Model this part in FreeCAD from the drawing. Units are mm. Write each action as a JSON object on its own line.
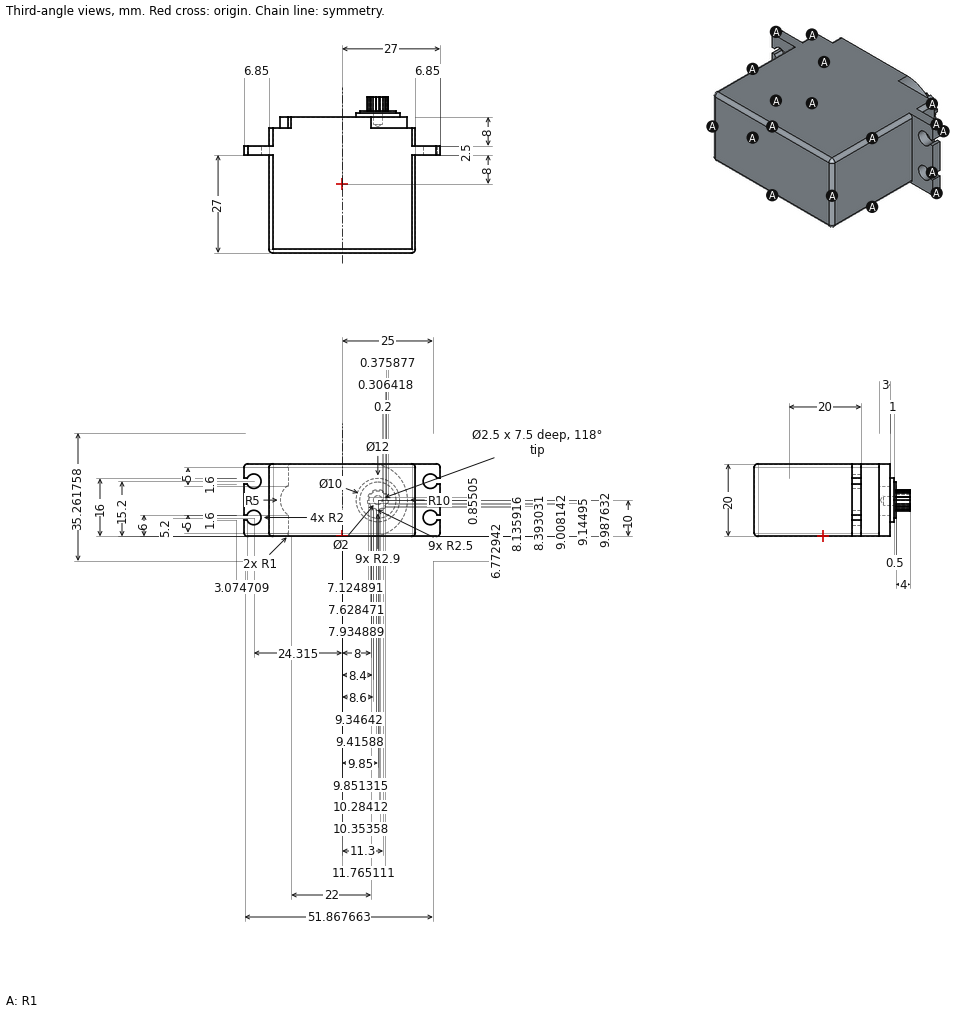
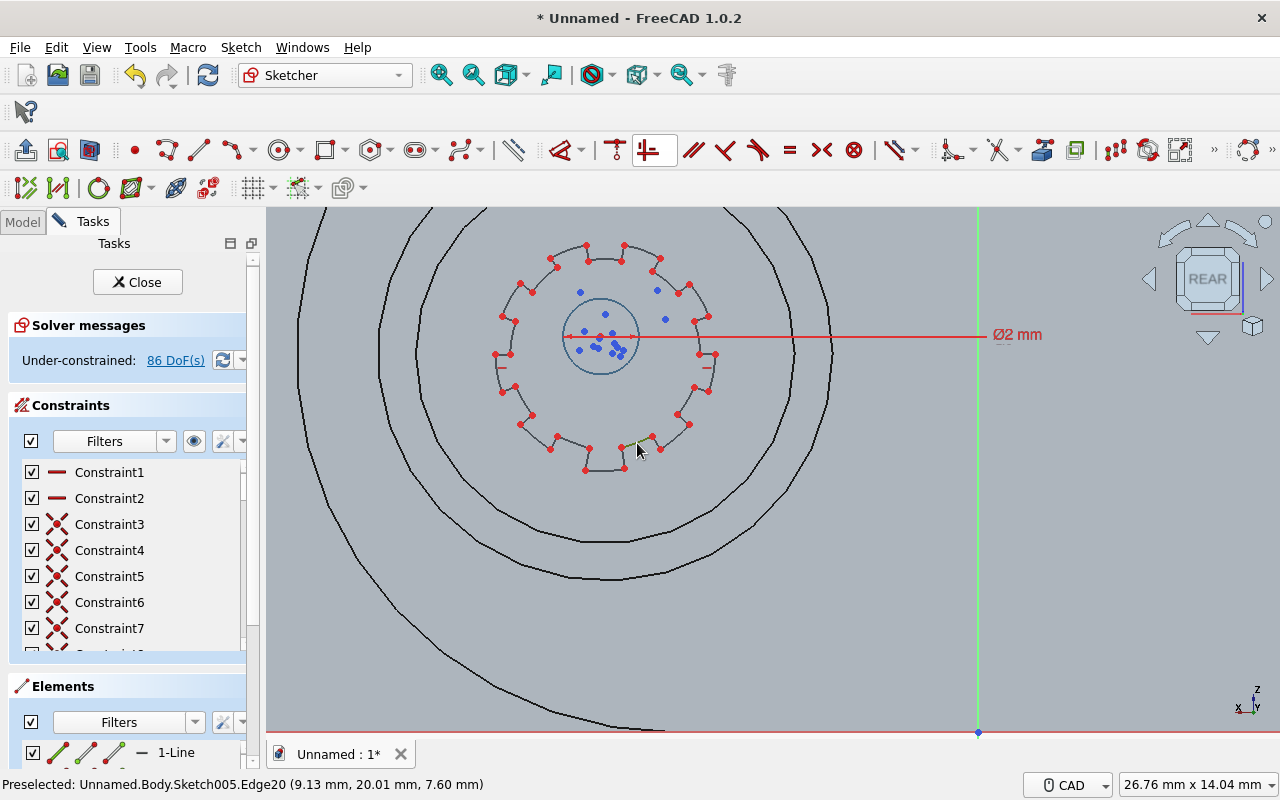
{"action": "left_click", "coordinate": [616, 150]}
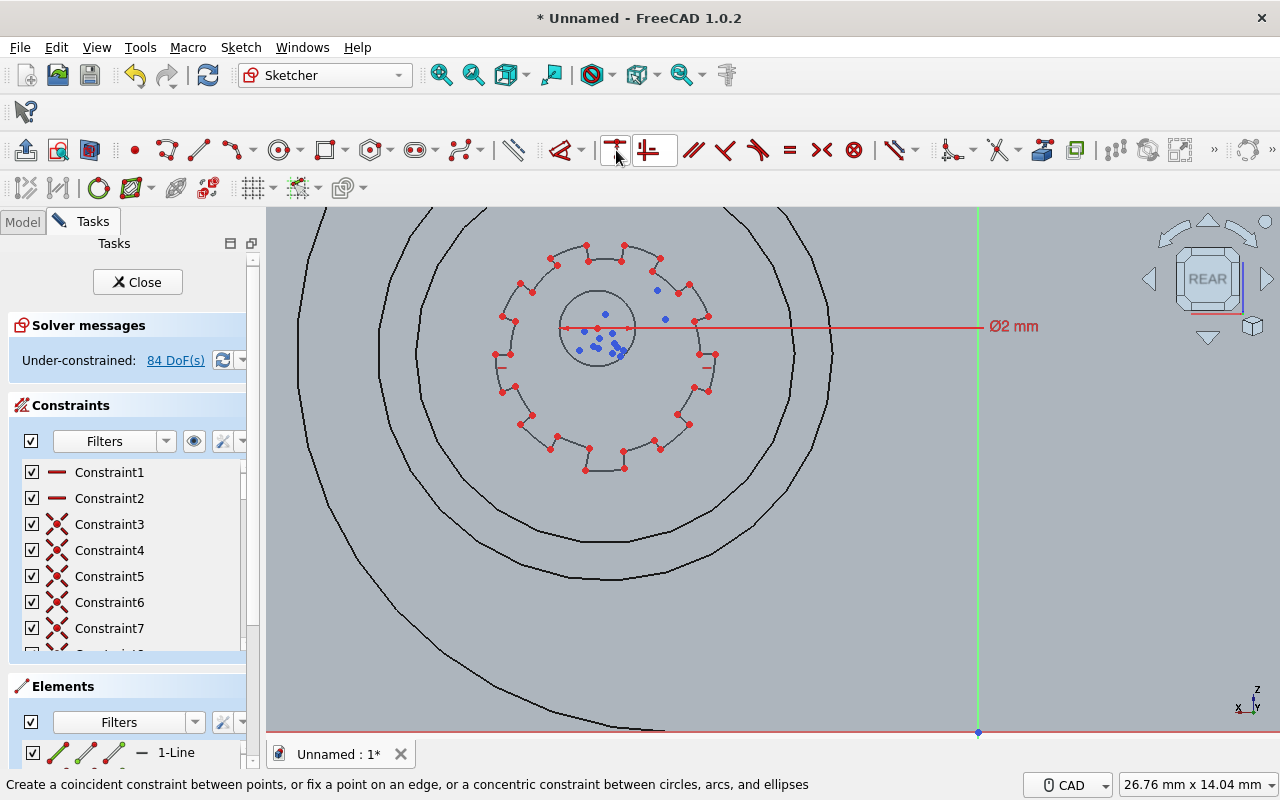
{"action": "left_click", "coordinate": [624, 302]}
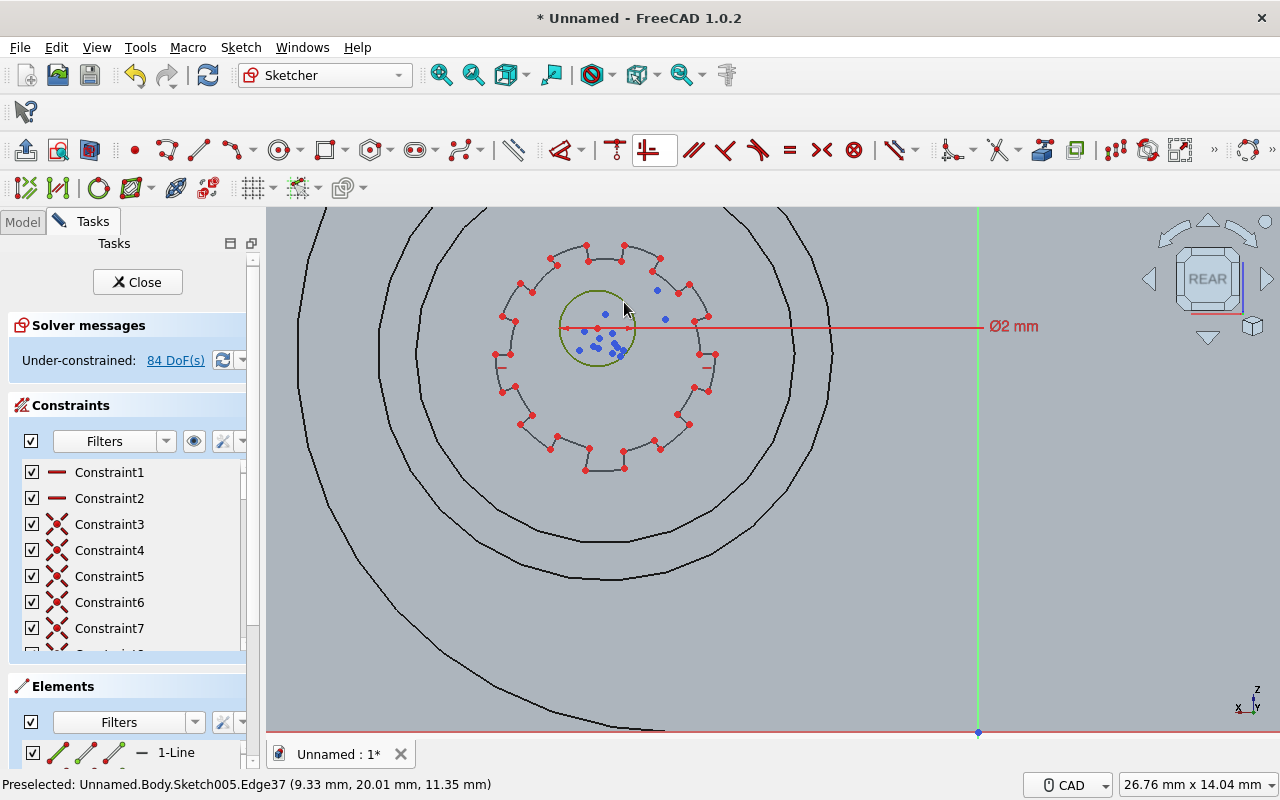
{"action": "left_click", "coordinate": [670, 443]}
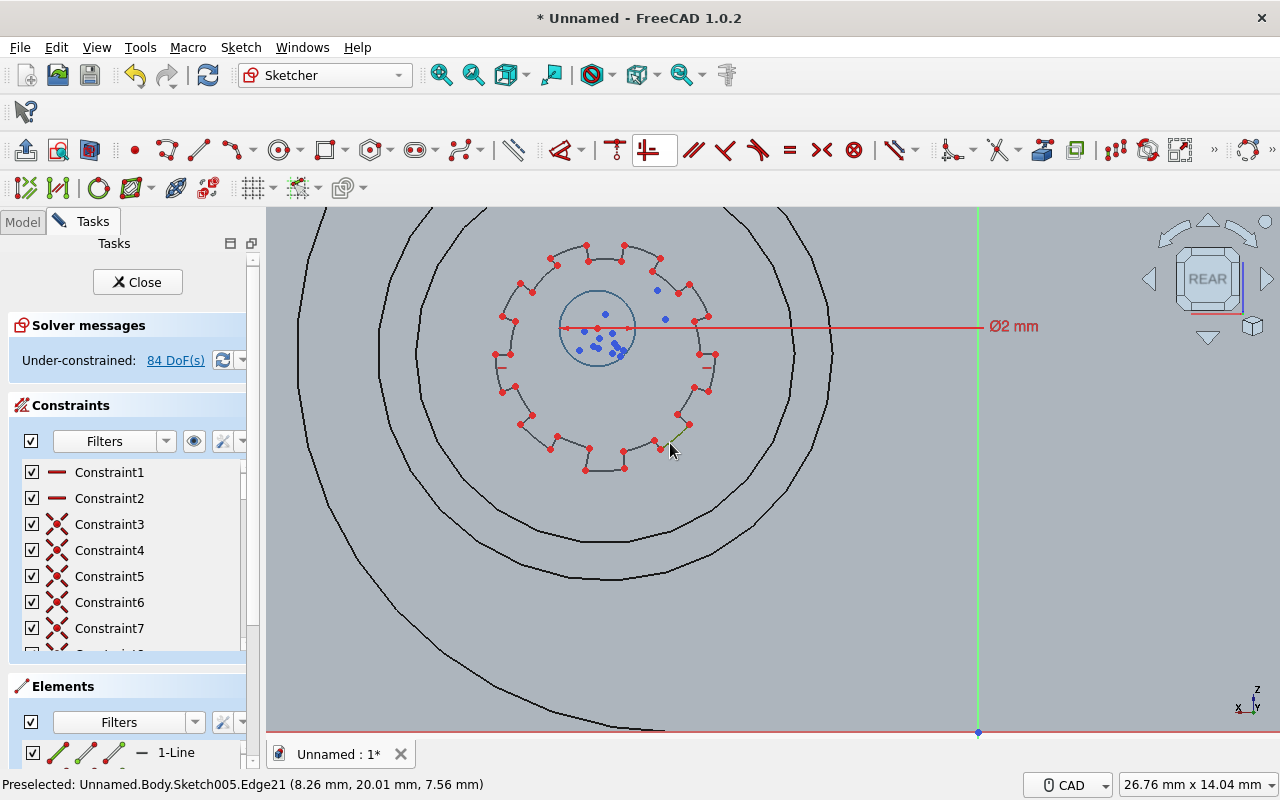
{"action": "left_click", "coordinate": [616, 150]}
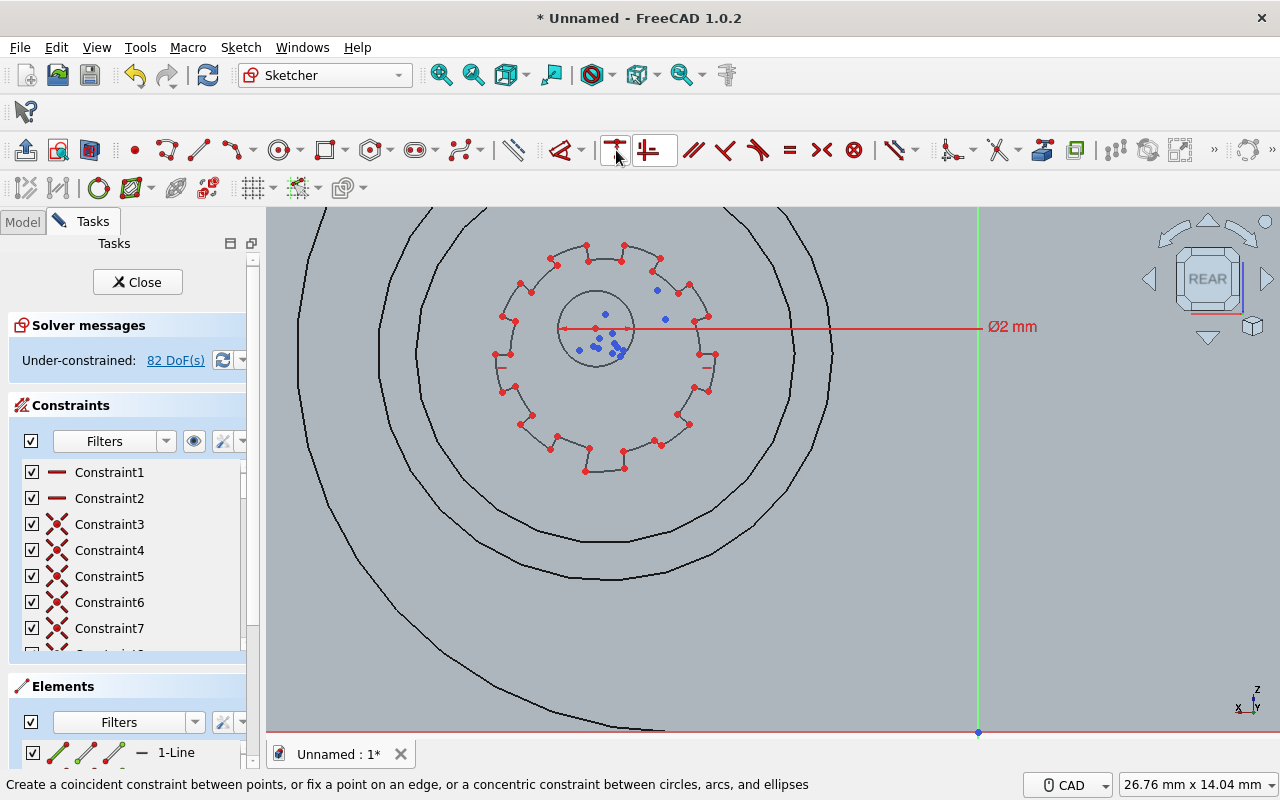
{"action": "left_click", "coordinate": [623, 302]}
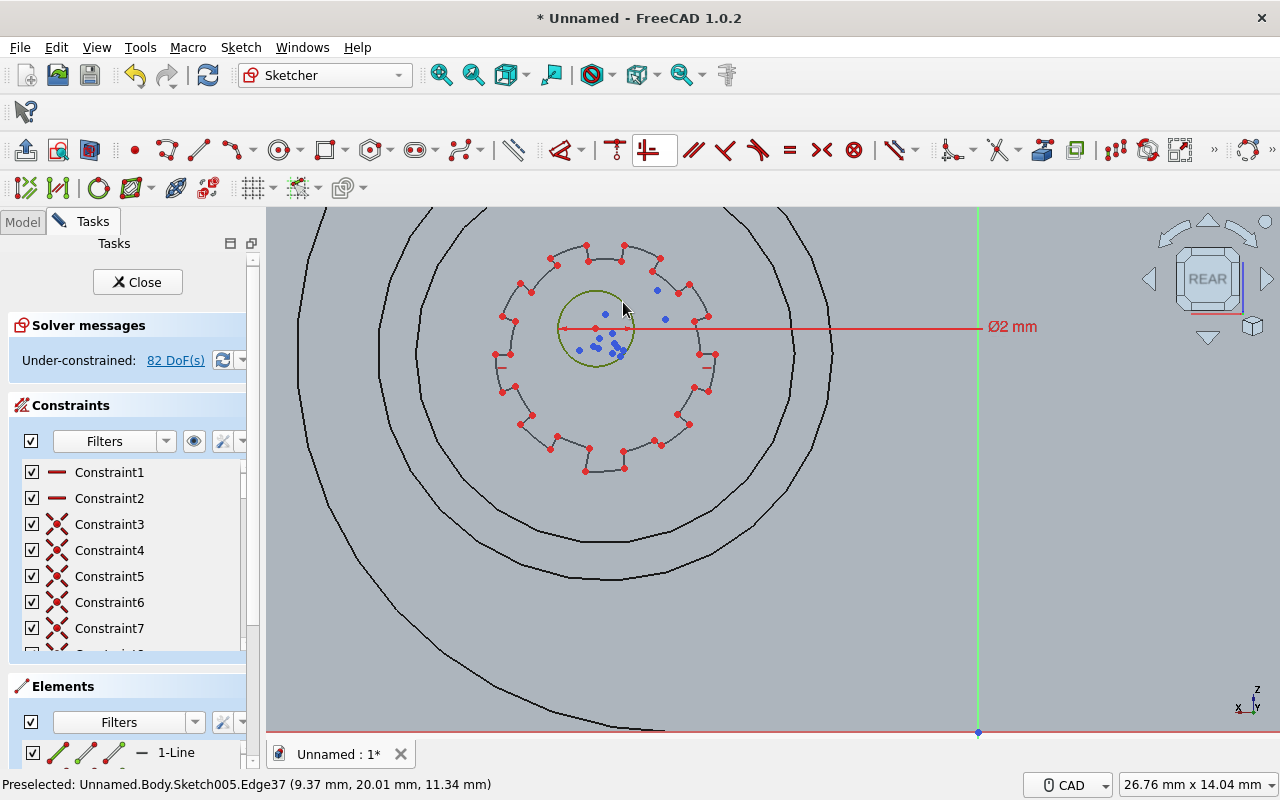
{"action": "scroll", "coordinate": [683, 407], "scroll_direction": "up", "scroll_amount": 2}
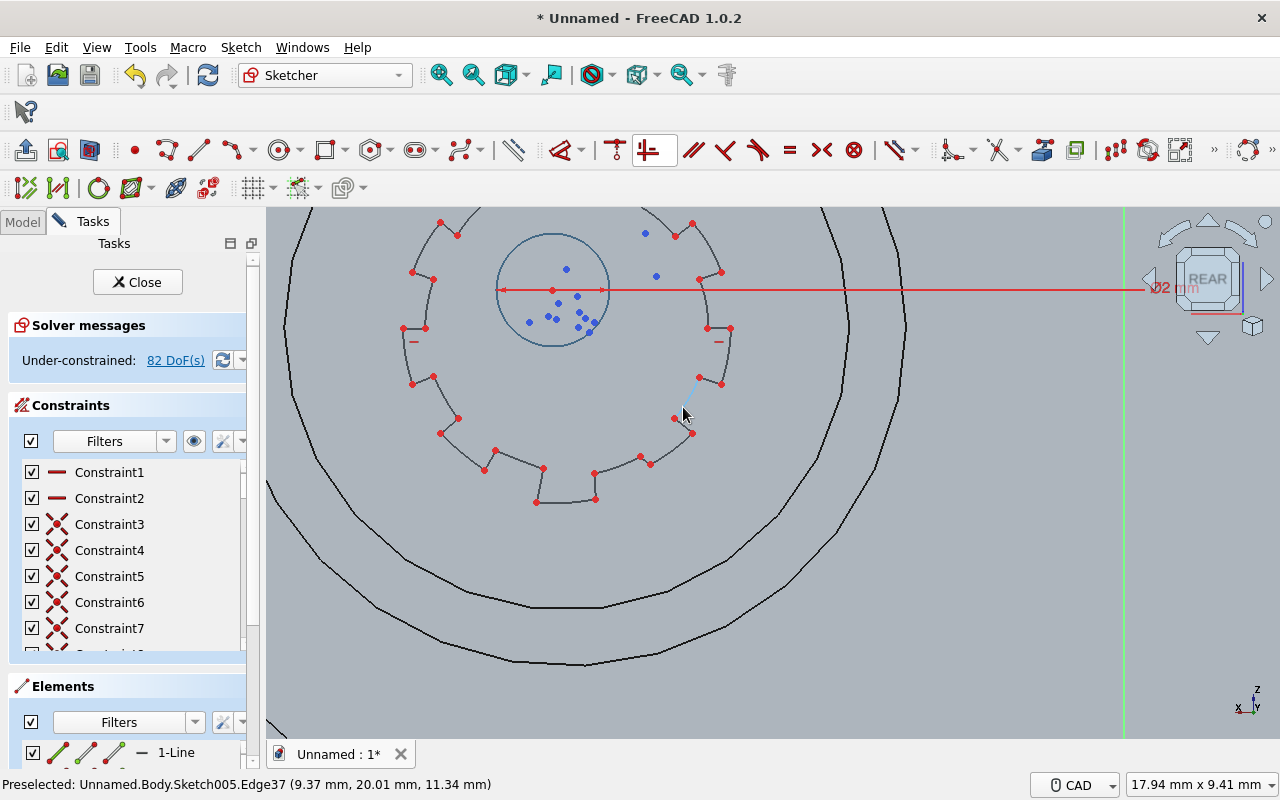
{"action": "left_click", "coordinate": [683, 407]}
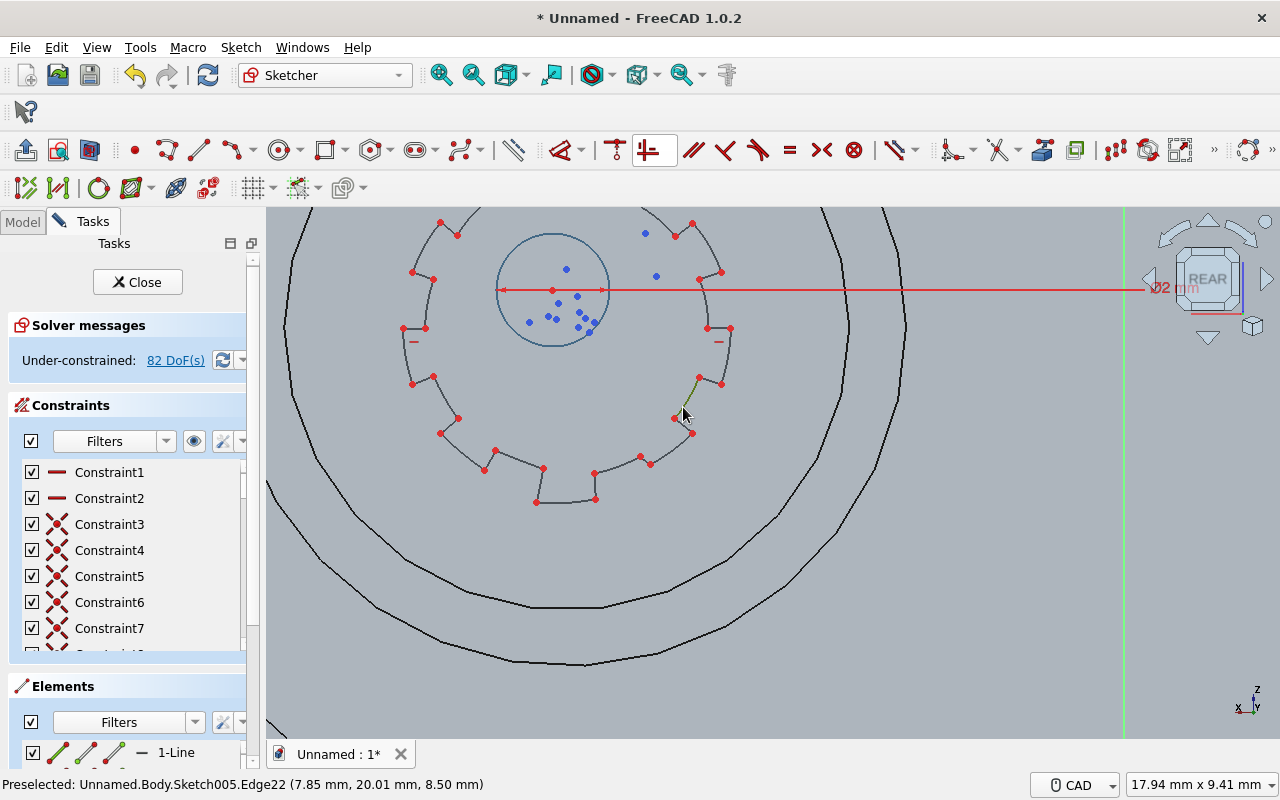
{"action": "left_click", "coordinate": [616, 150]}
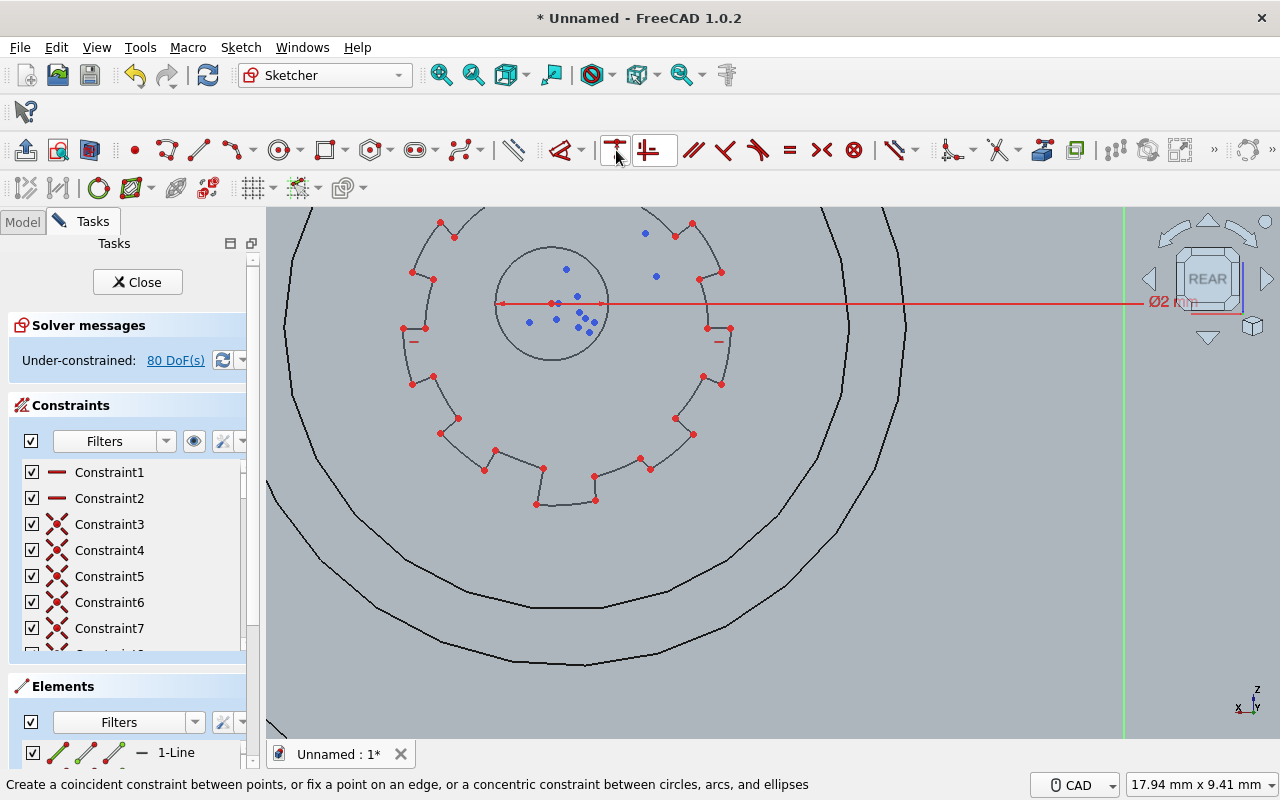
{"action": "left_click", "coordinate": [592, 264]}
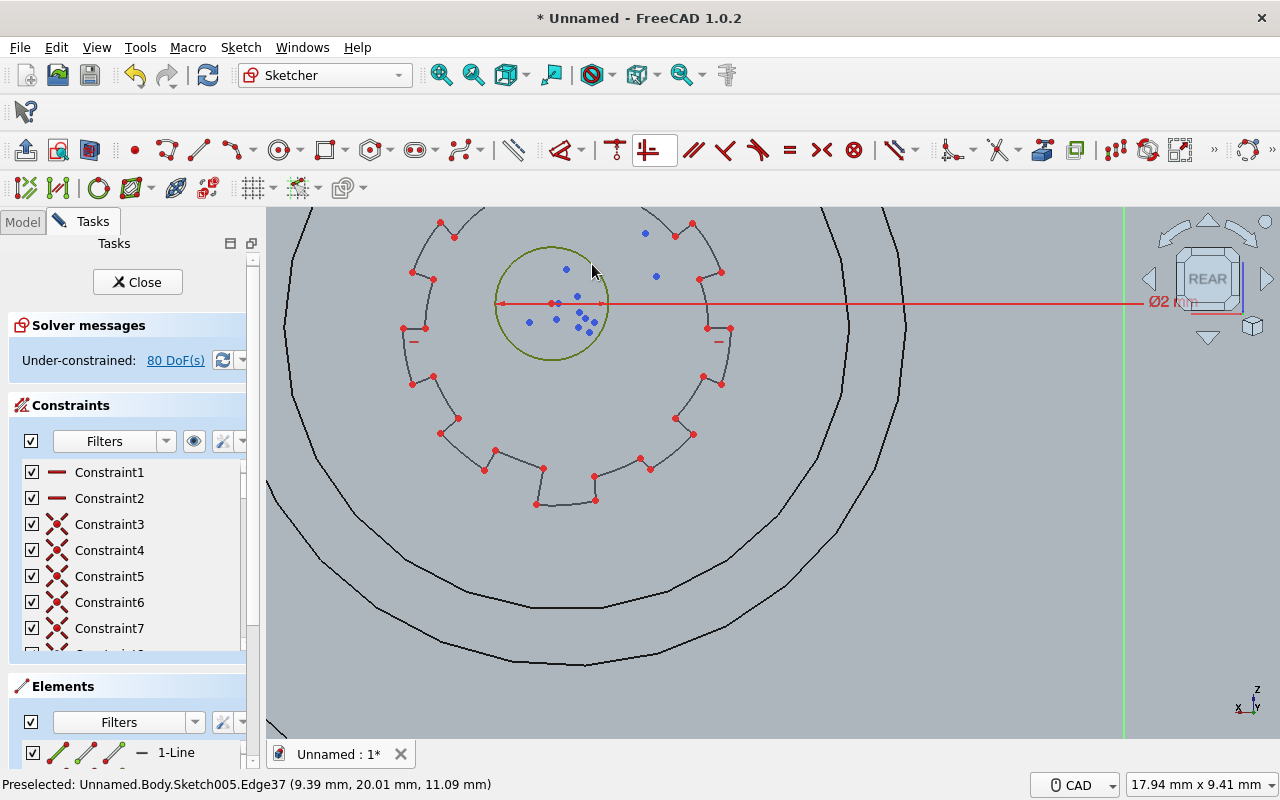
{"action": "left_click", "coordinate": [726, 368]}